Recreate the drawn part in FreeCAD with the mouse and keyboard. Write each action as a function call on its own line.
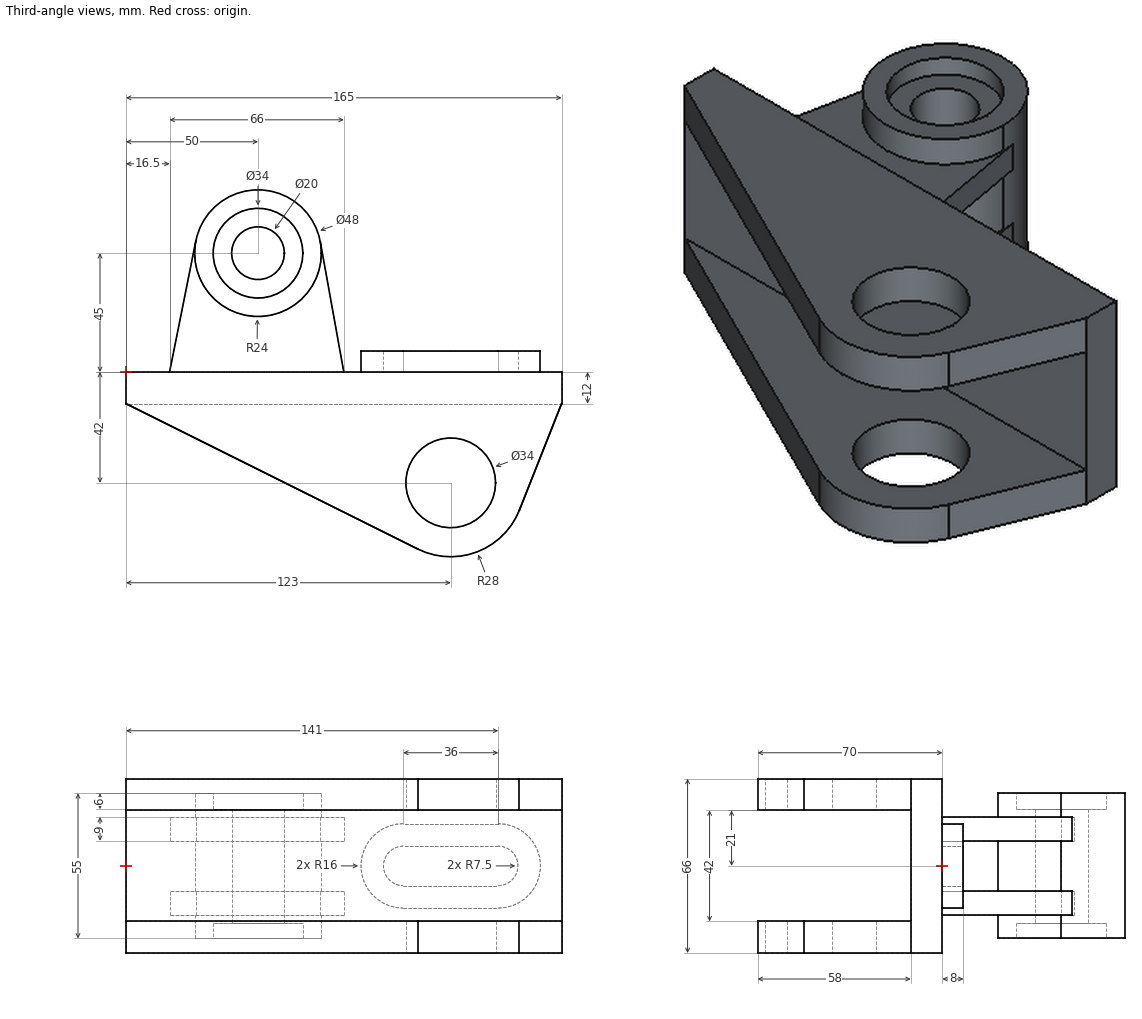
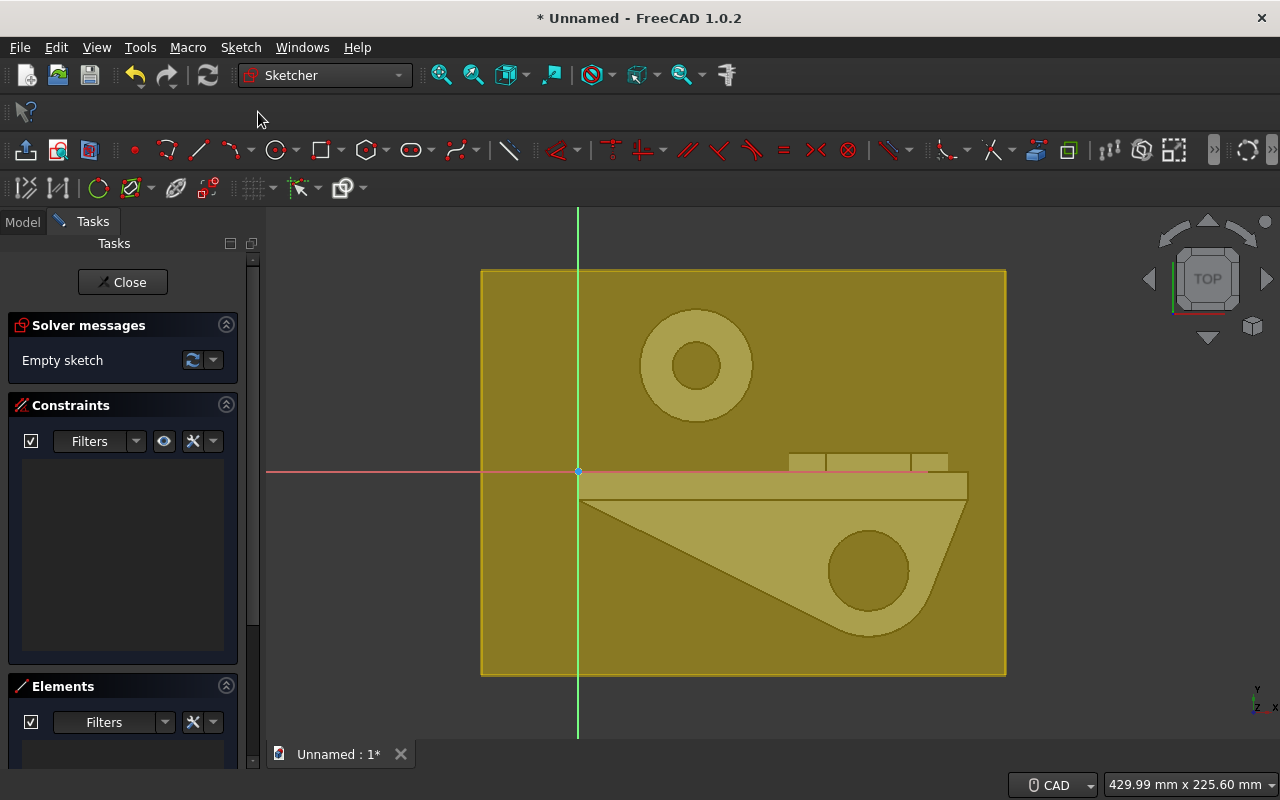
scroll(659, 378, up, 5)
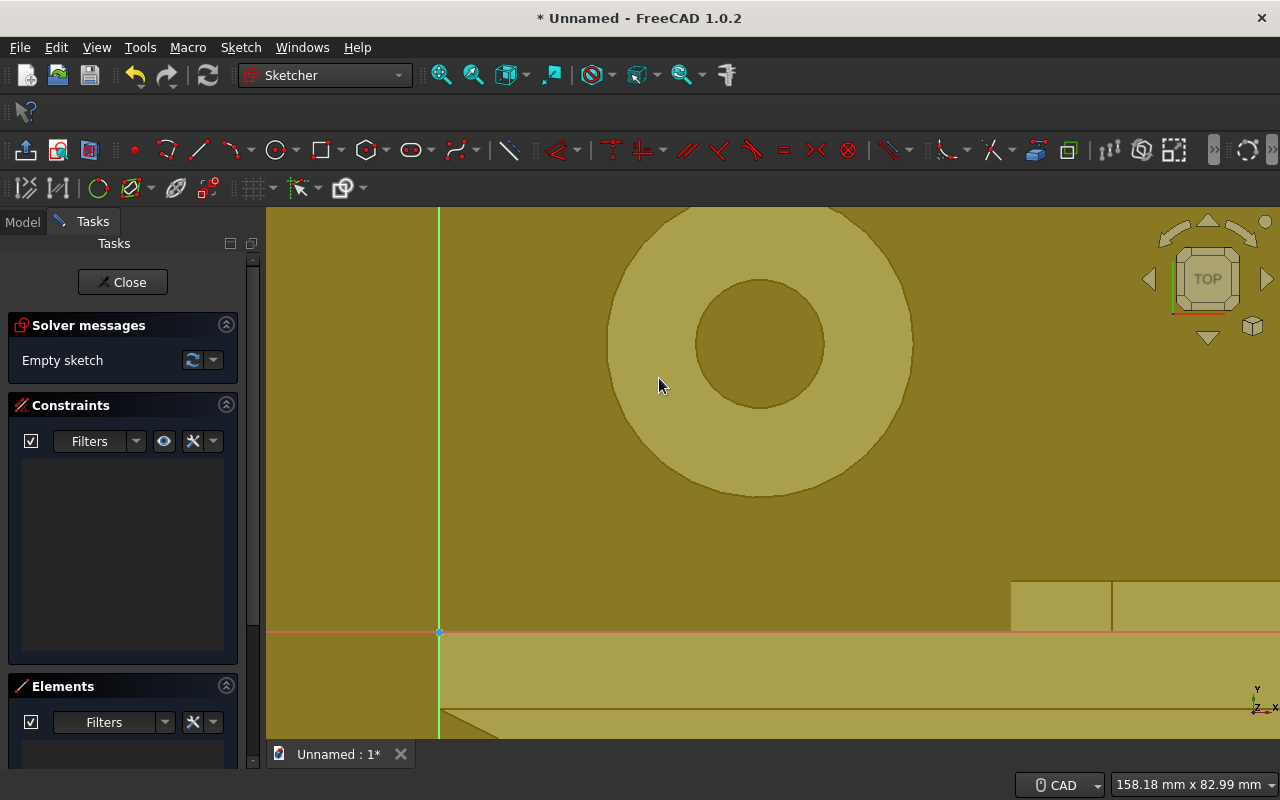
key(g)
key(m)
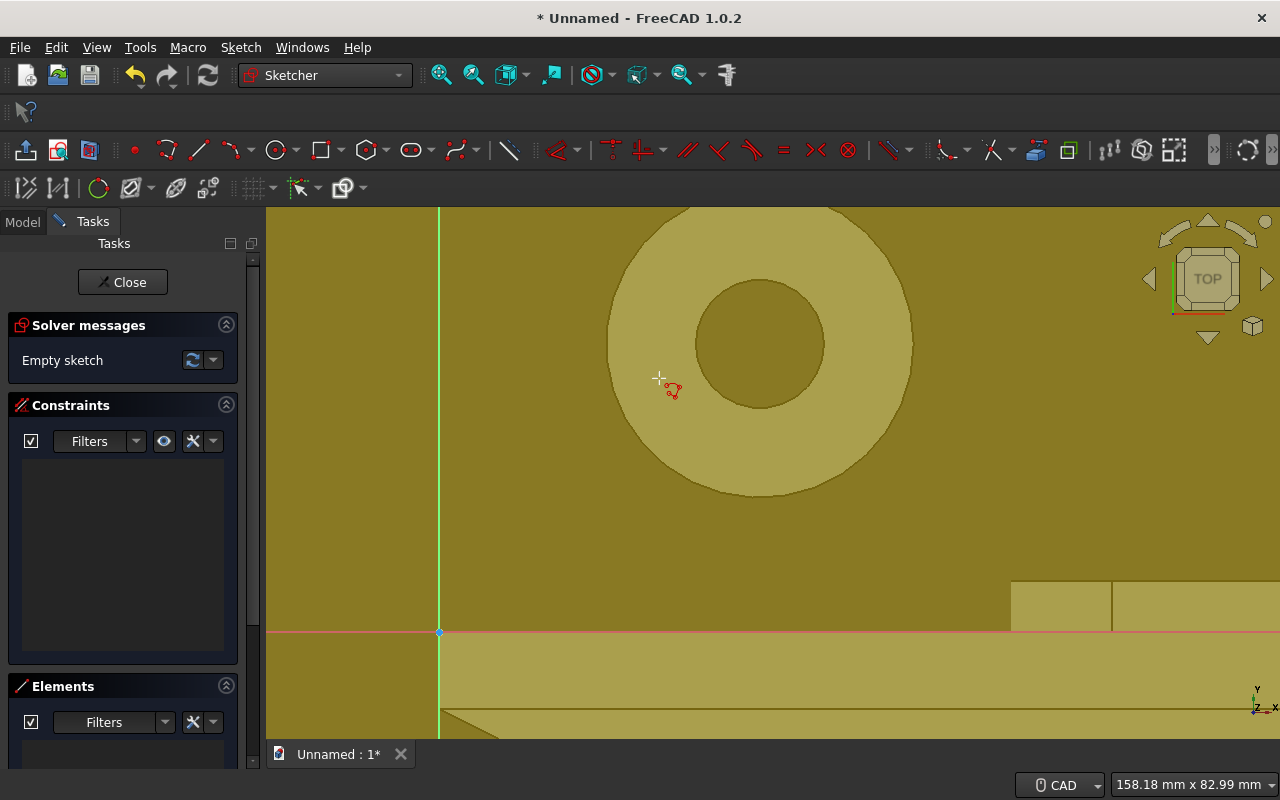
click(609, 314)
click(545, 632)
click(968, 623)
click(911, 317)
right_click(911, 317)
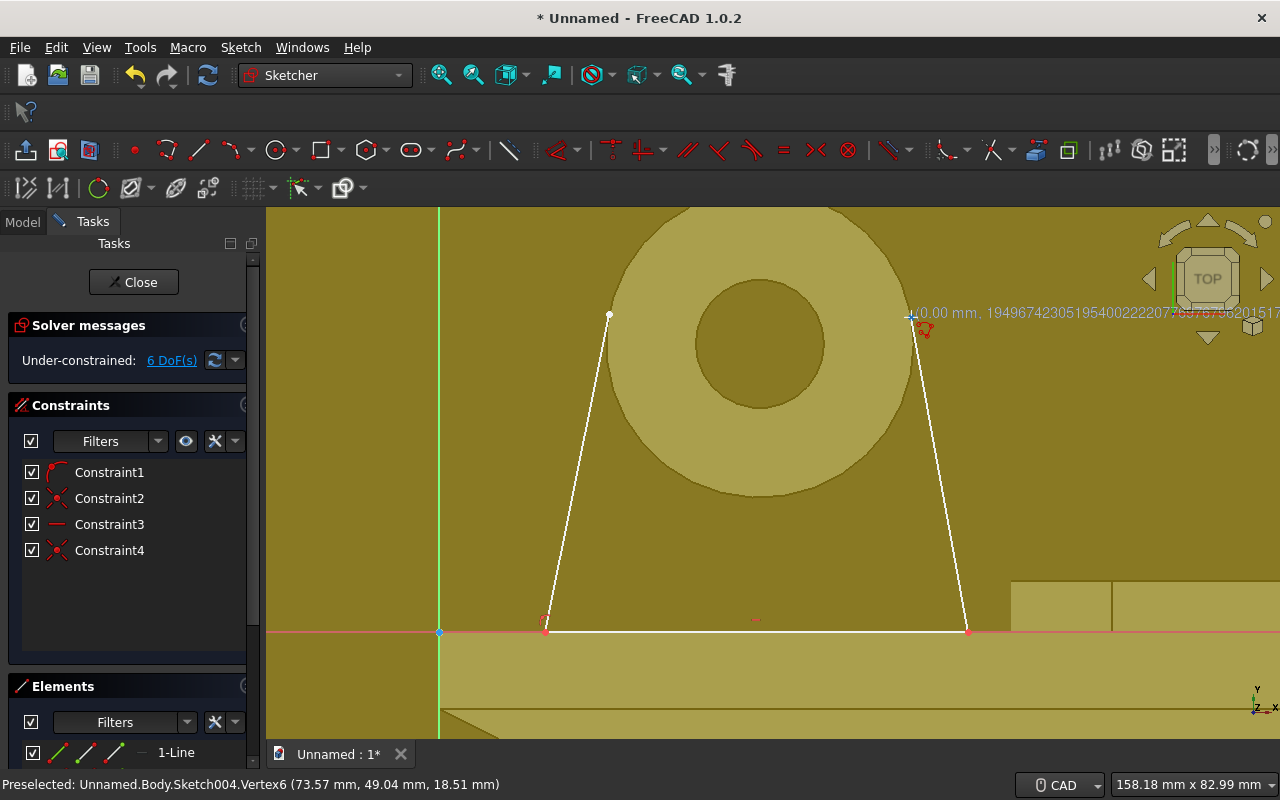
key(g)
key(3)
key(a)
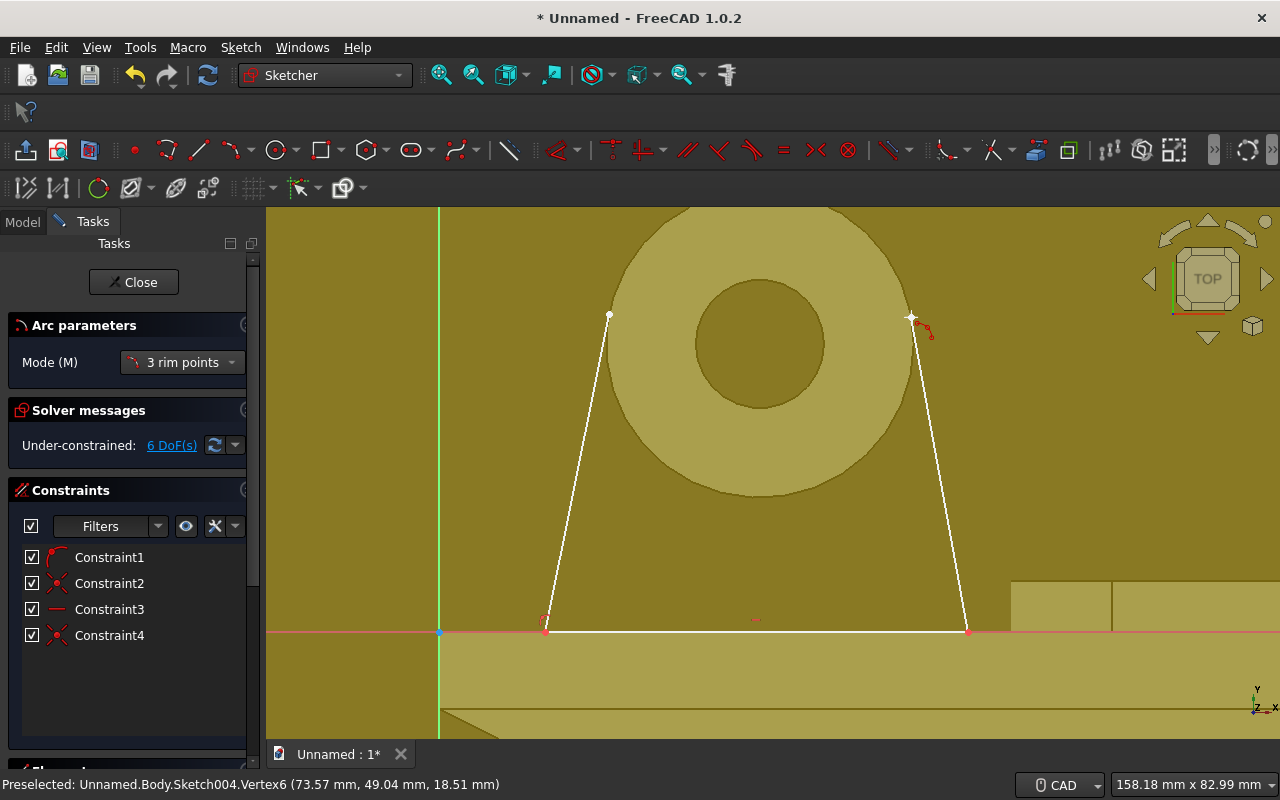
click(911, 318)
click(609, 315)
click(758, 498)
key(Escape)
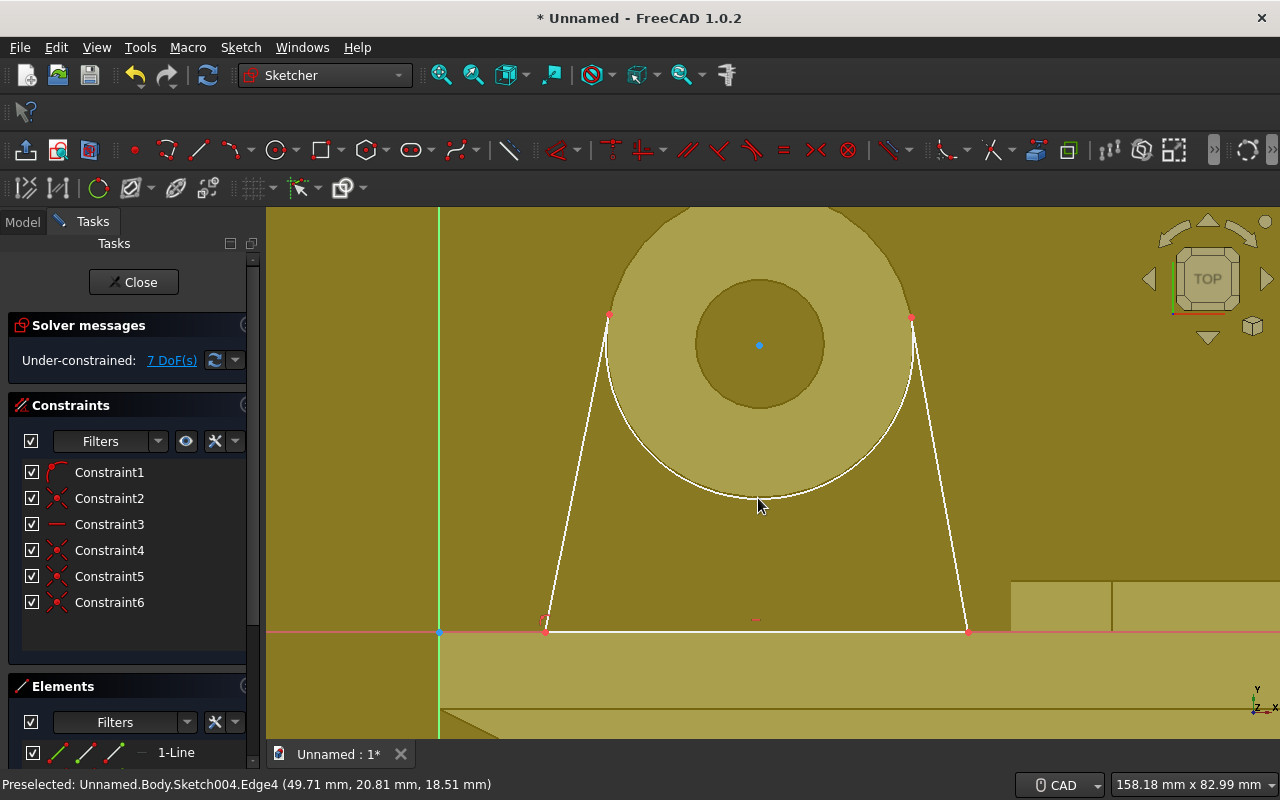
click(590, 410)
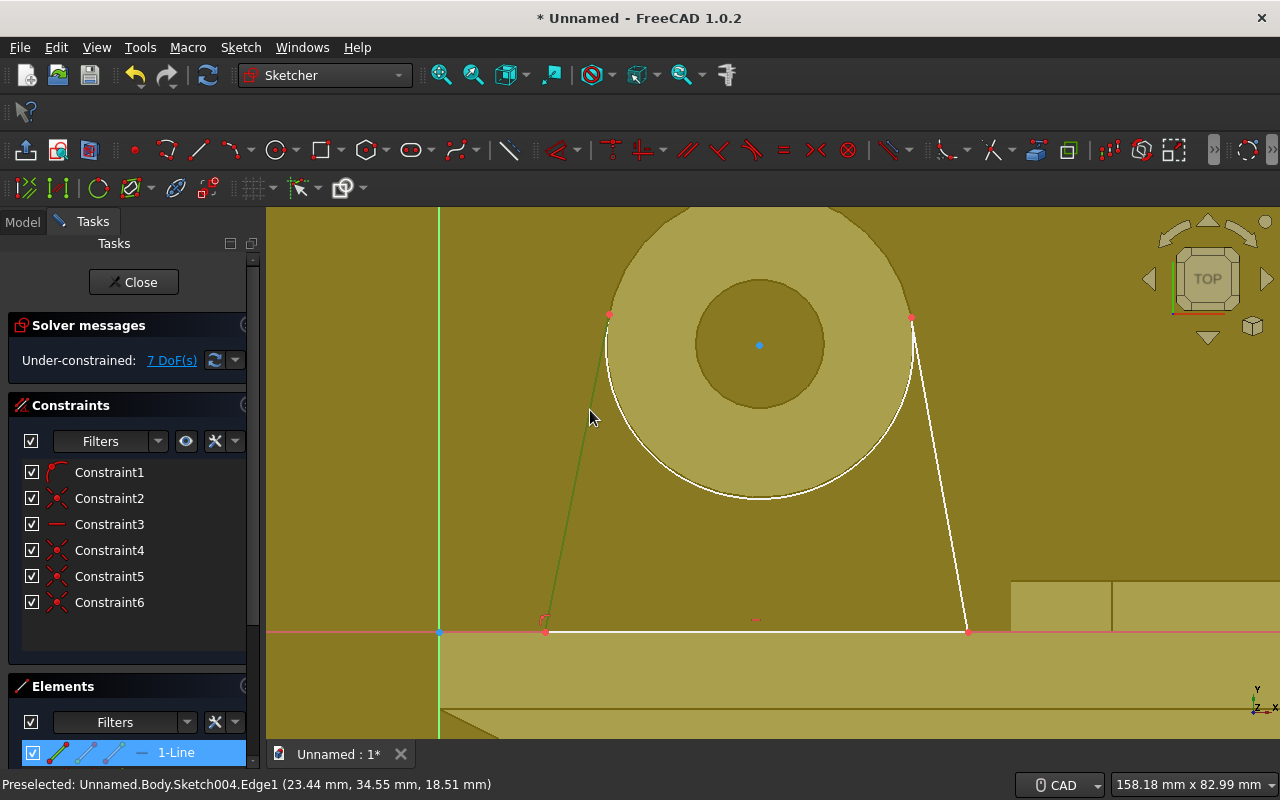
click(659, 462)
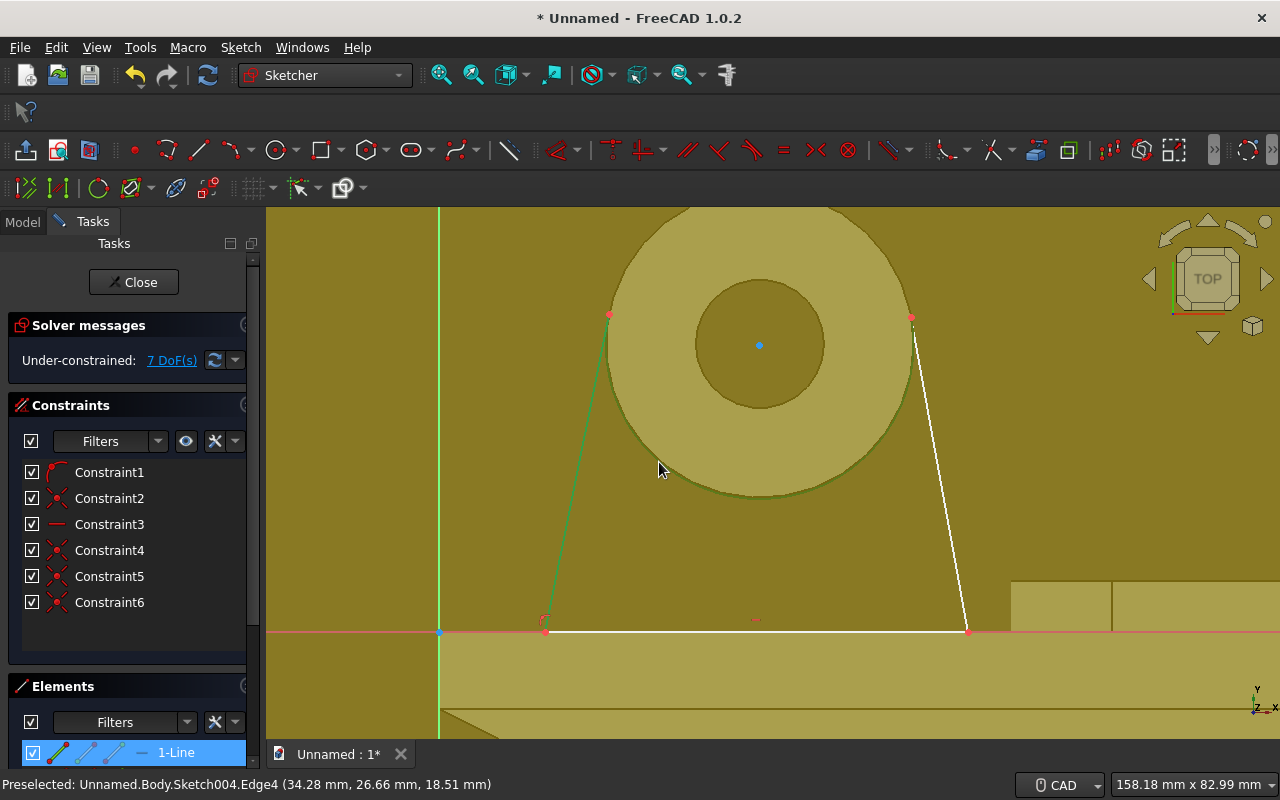
key(t)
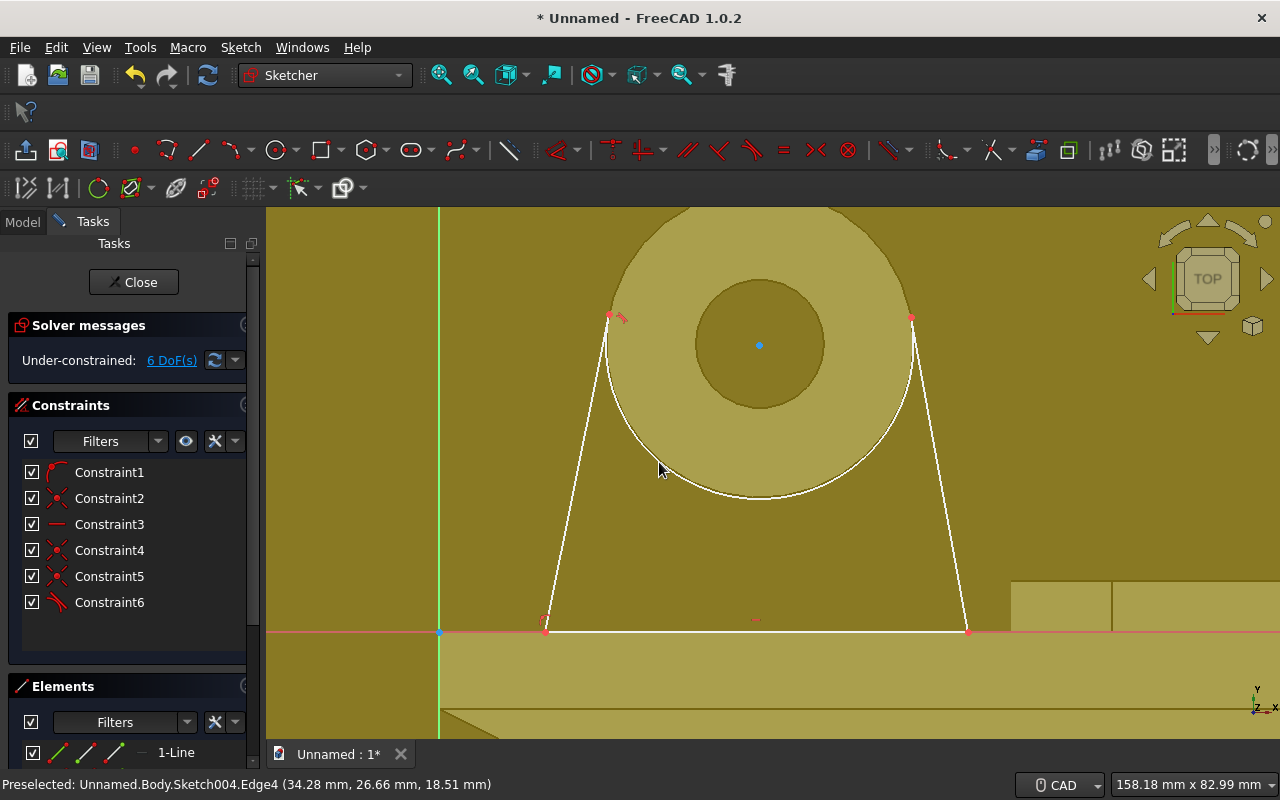
click(951, 538)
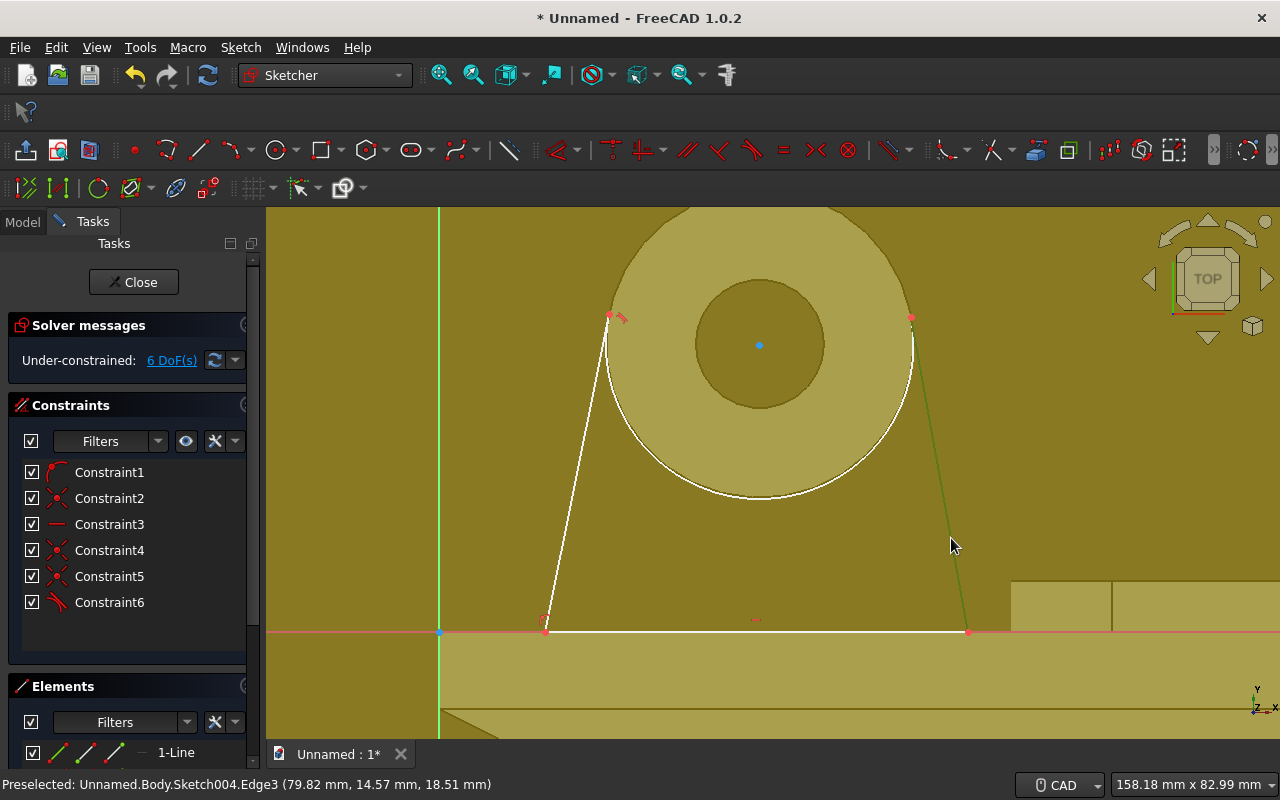
click(659, 461)